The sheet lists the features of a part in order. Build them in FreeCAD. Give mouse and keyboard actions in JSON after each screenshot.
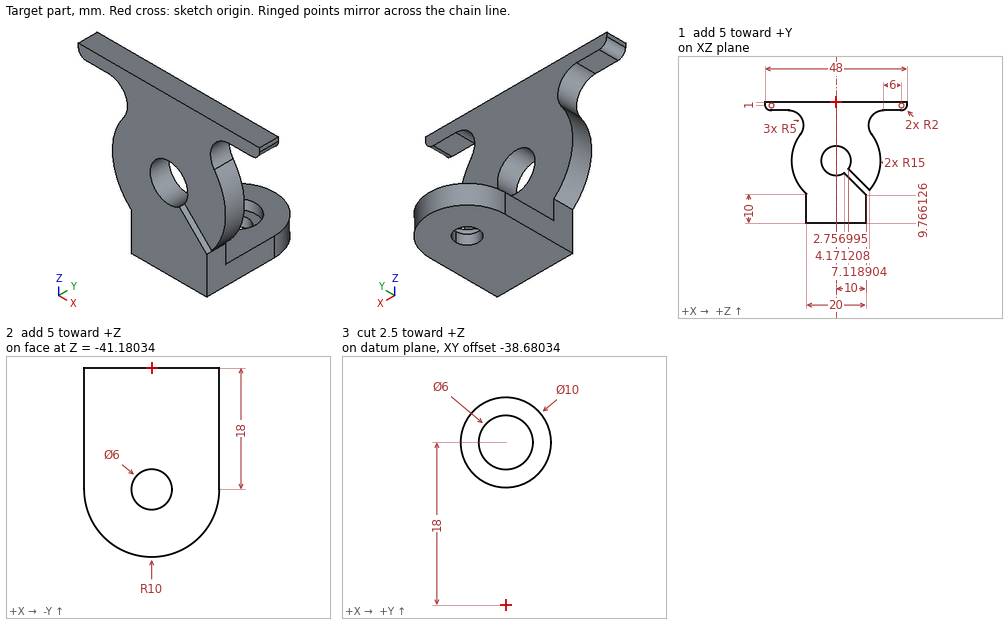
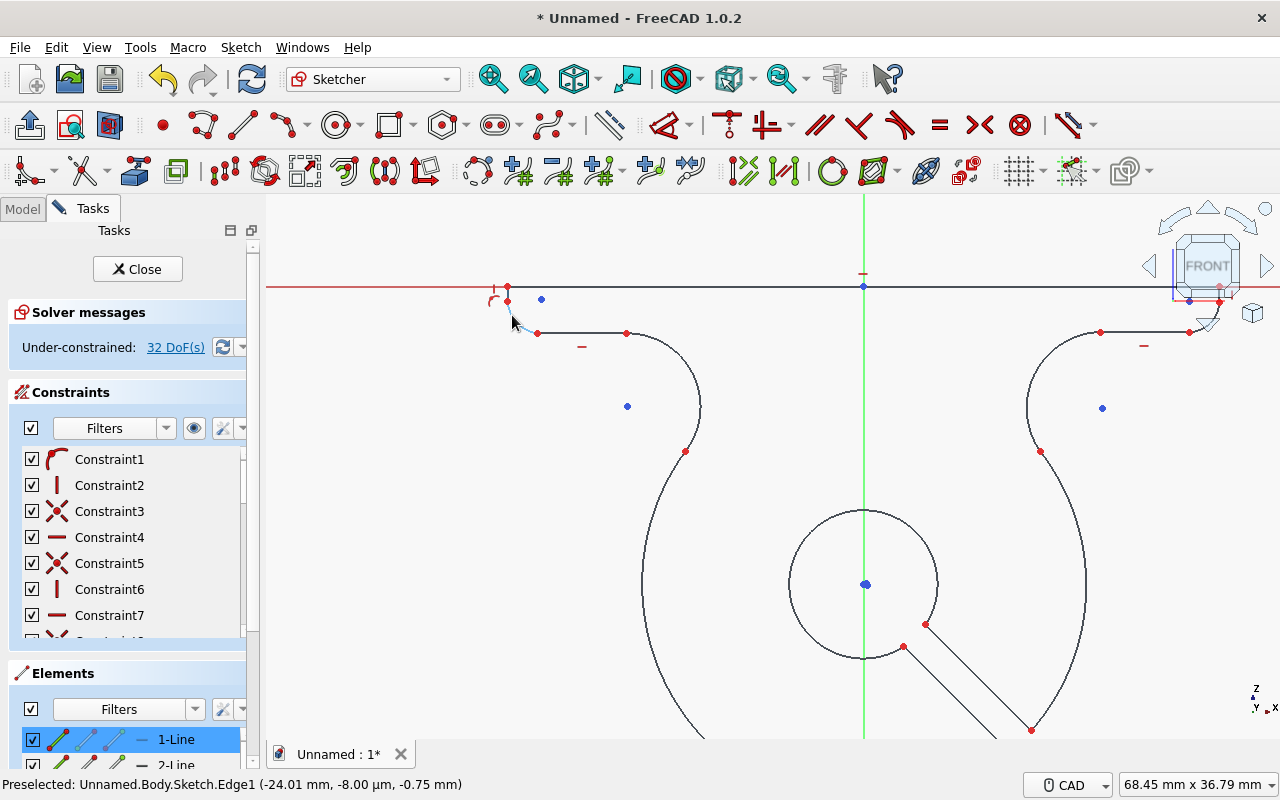
{"action": "left_click", "coordinate": [512, 315]}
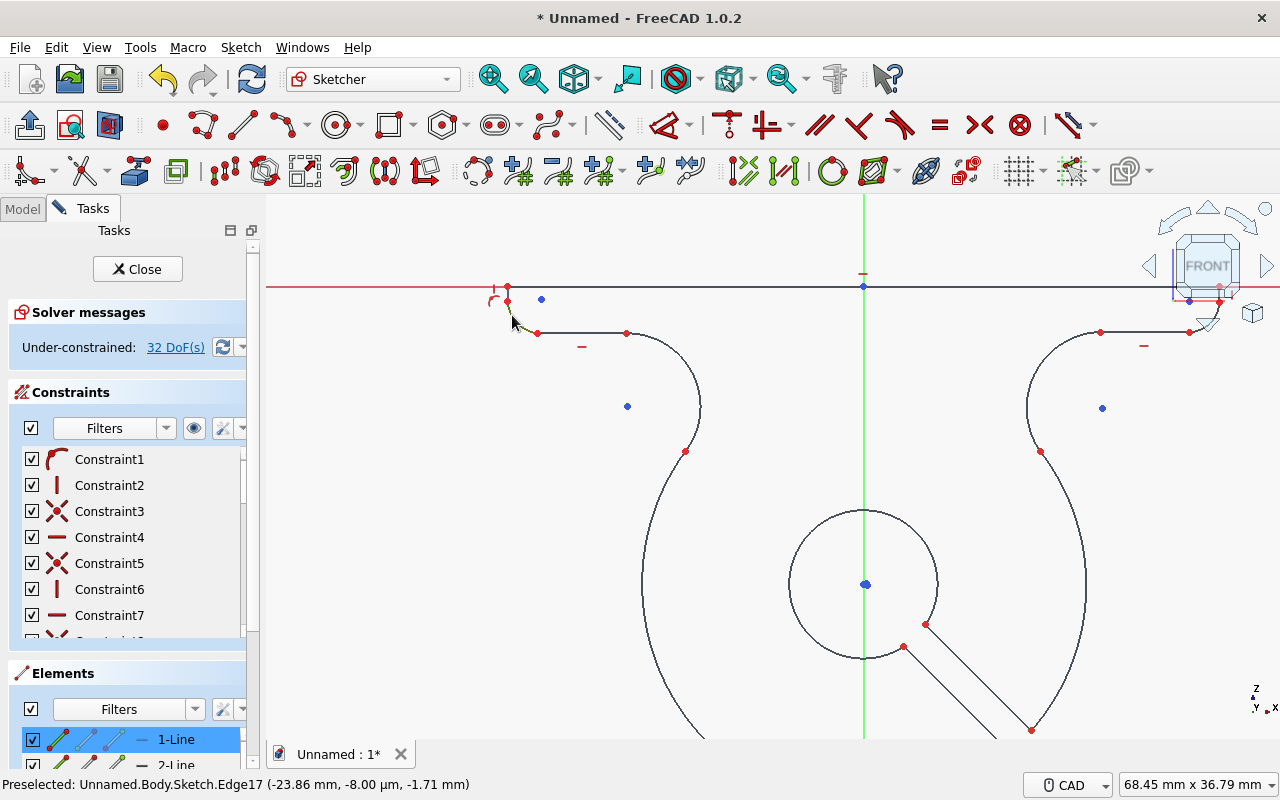
{"action": "key", "text": "t"}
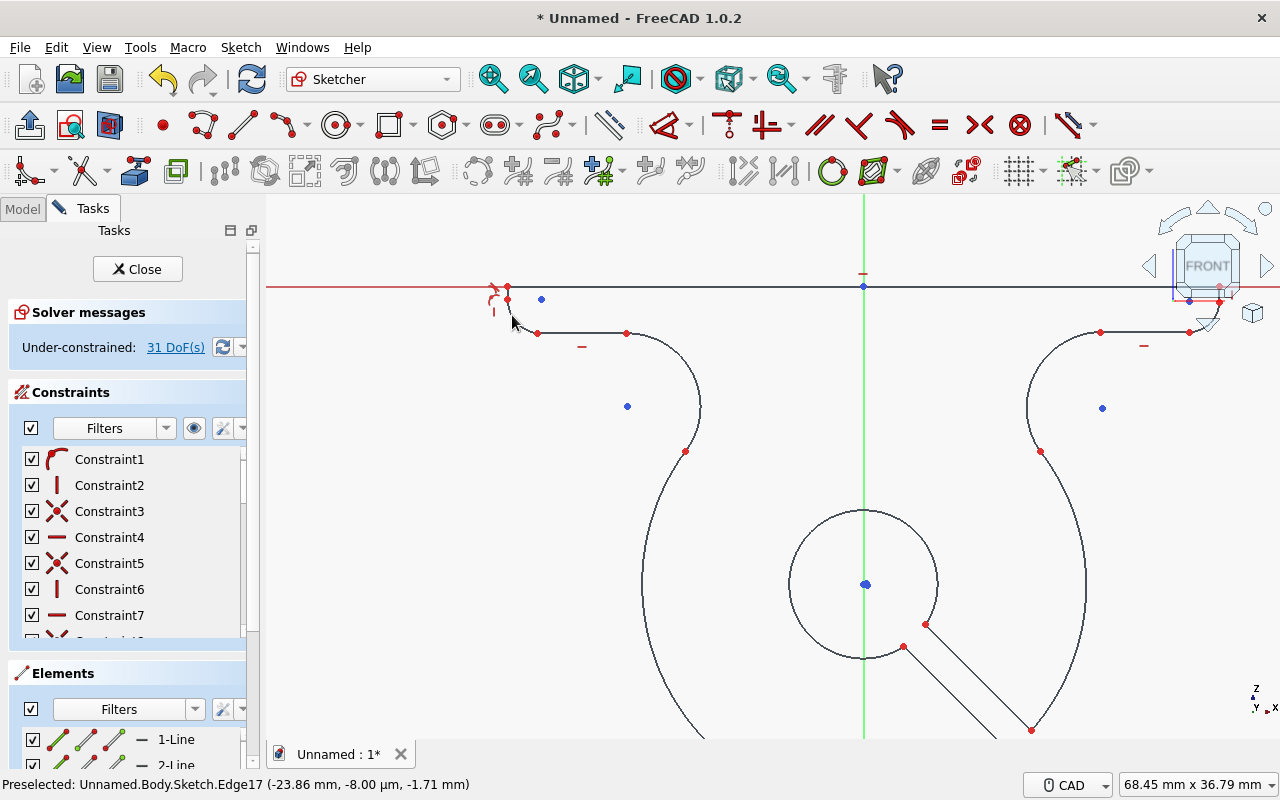
{"action": "scroll", "coordinate": [511, 314], "scroll_direction": "down", "scroll_amount": 3}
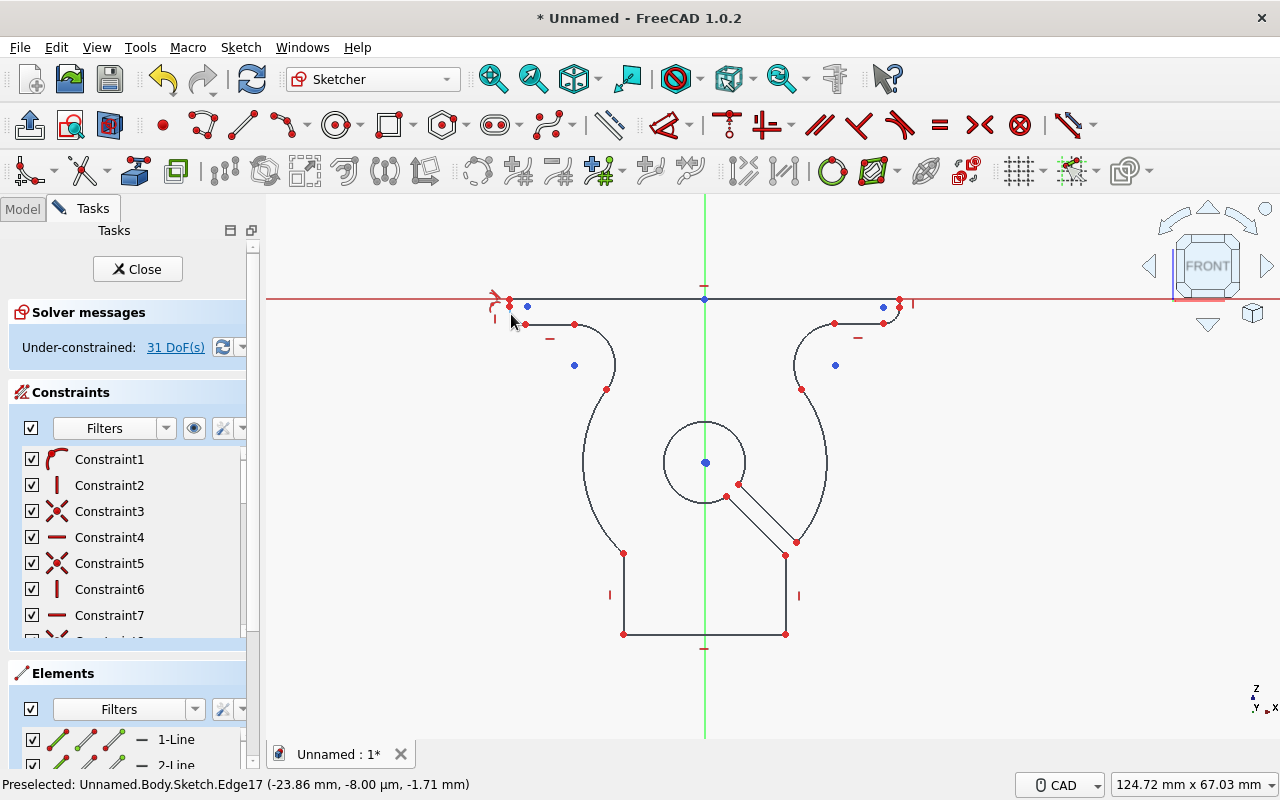
{"action": "scroll", "coordinate": [900, 303], "scroll_direction": "up", "scroll_amount": 6}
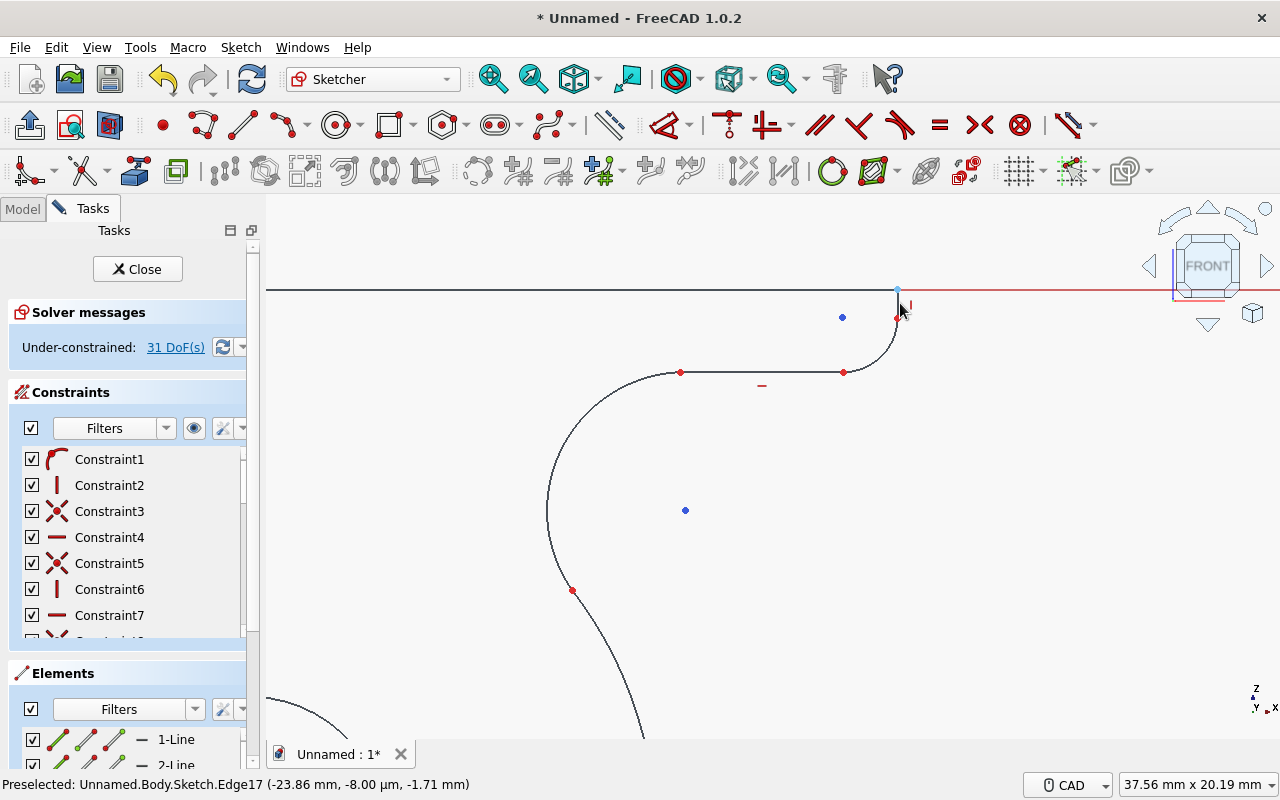
{"action": "left_click", "coordinate": [898, 304]}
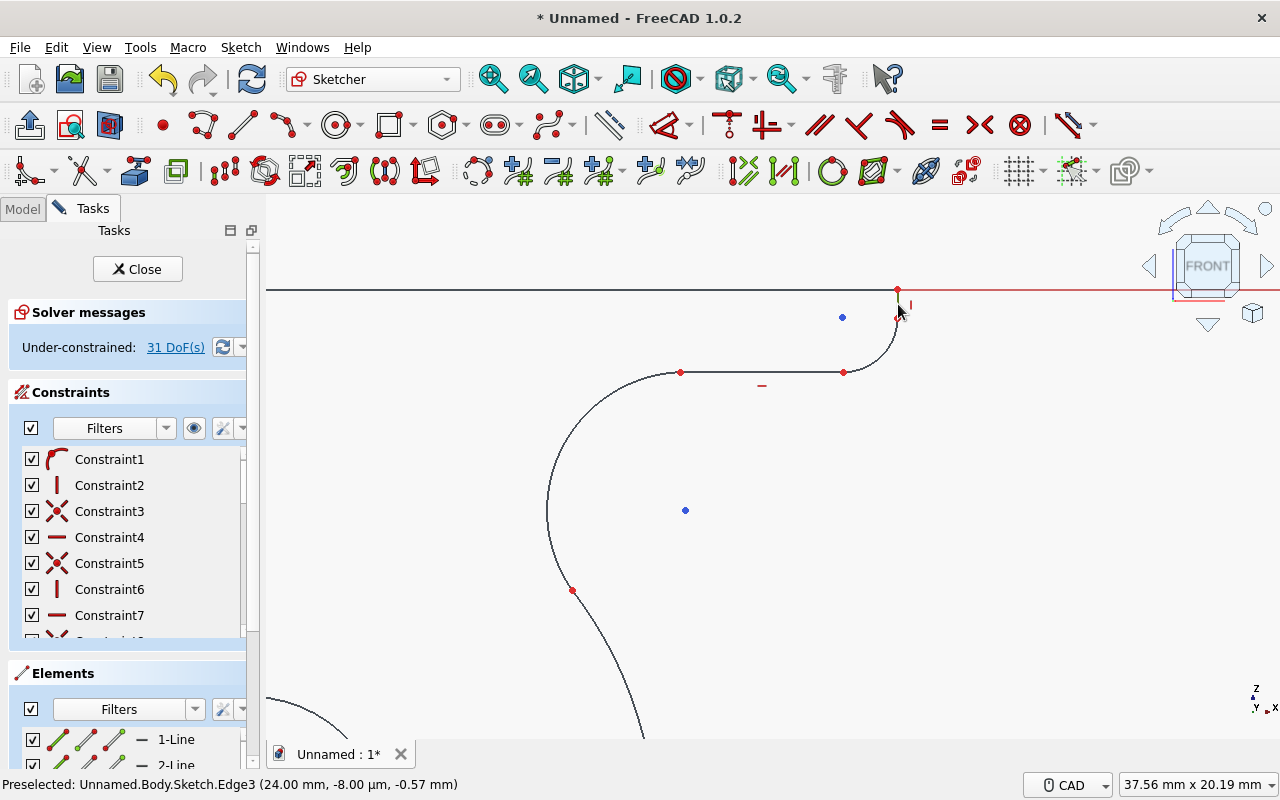
{"action": "left_click", "coordinate": [868, 366]}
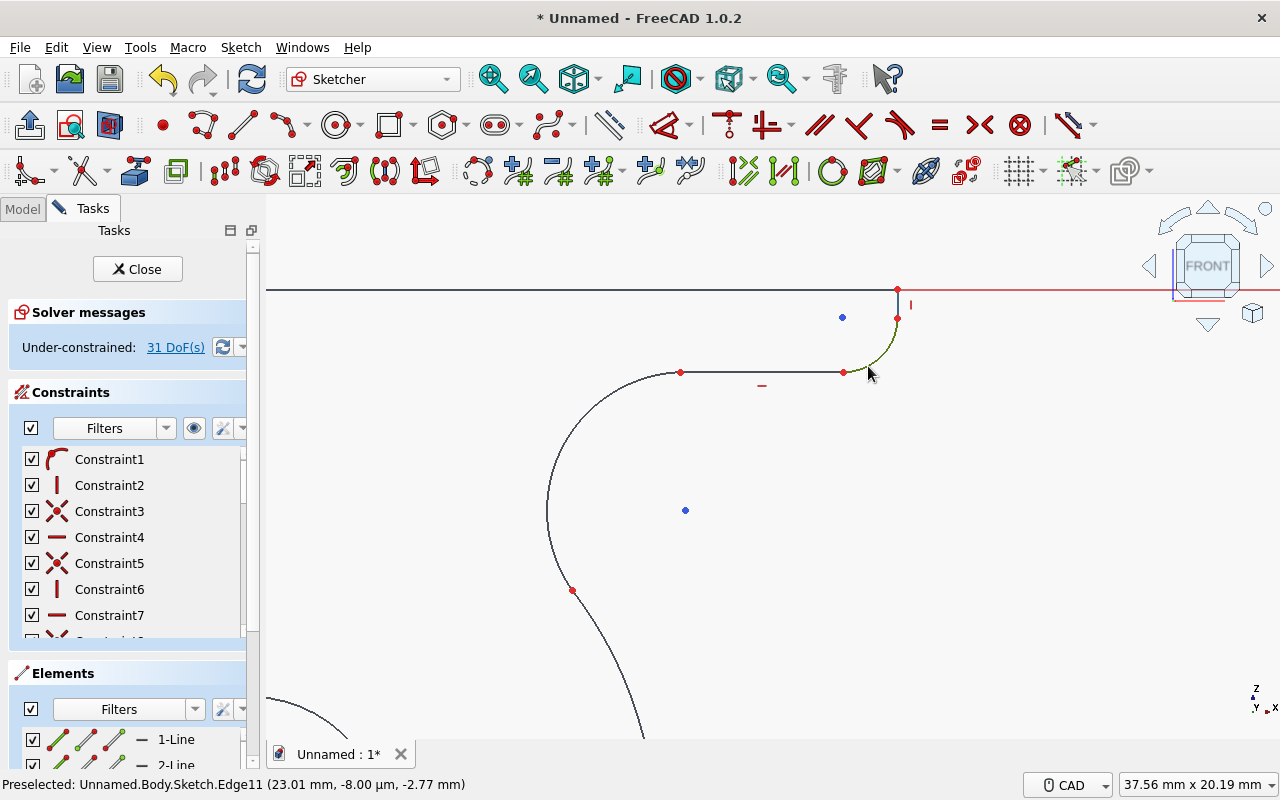
{"action": "key", "text": "t"}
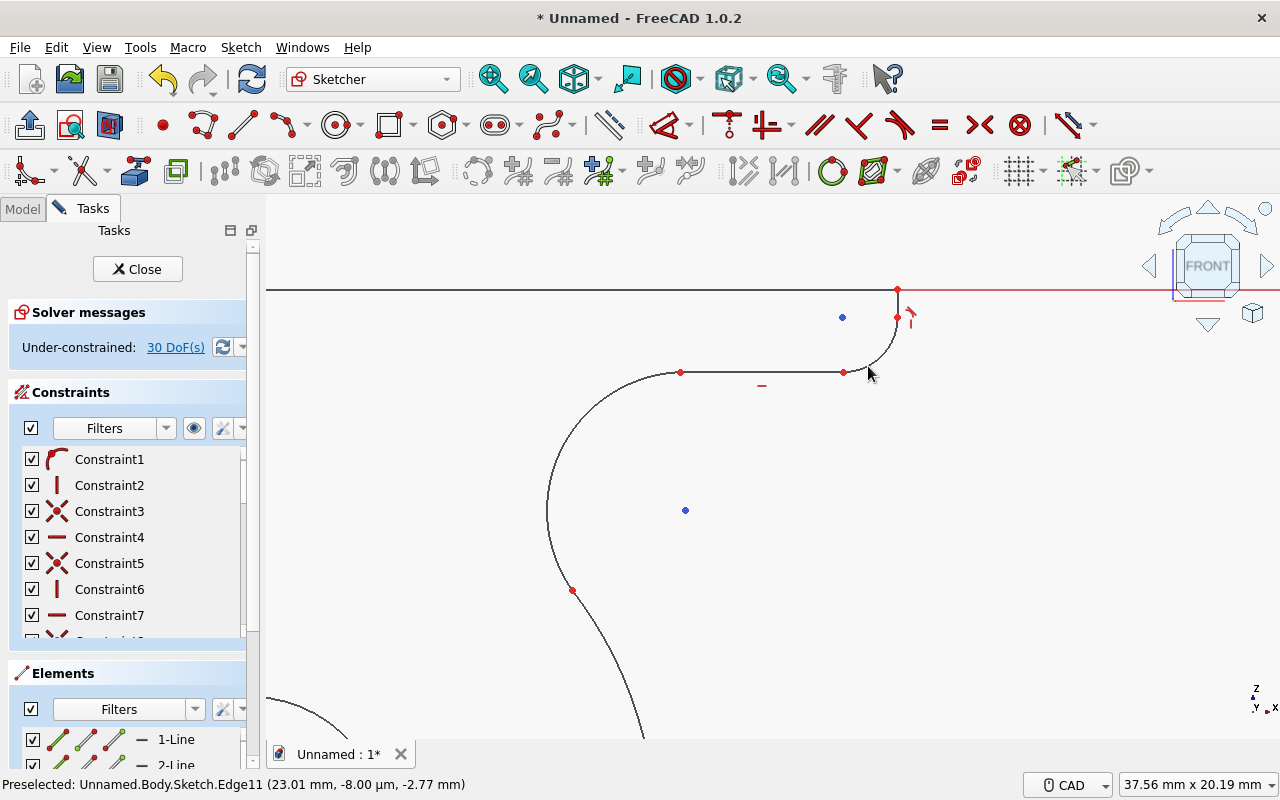
{"action": "left_click", "coordinate": [795, 372]}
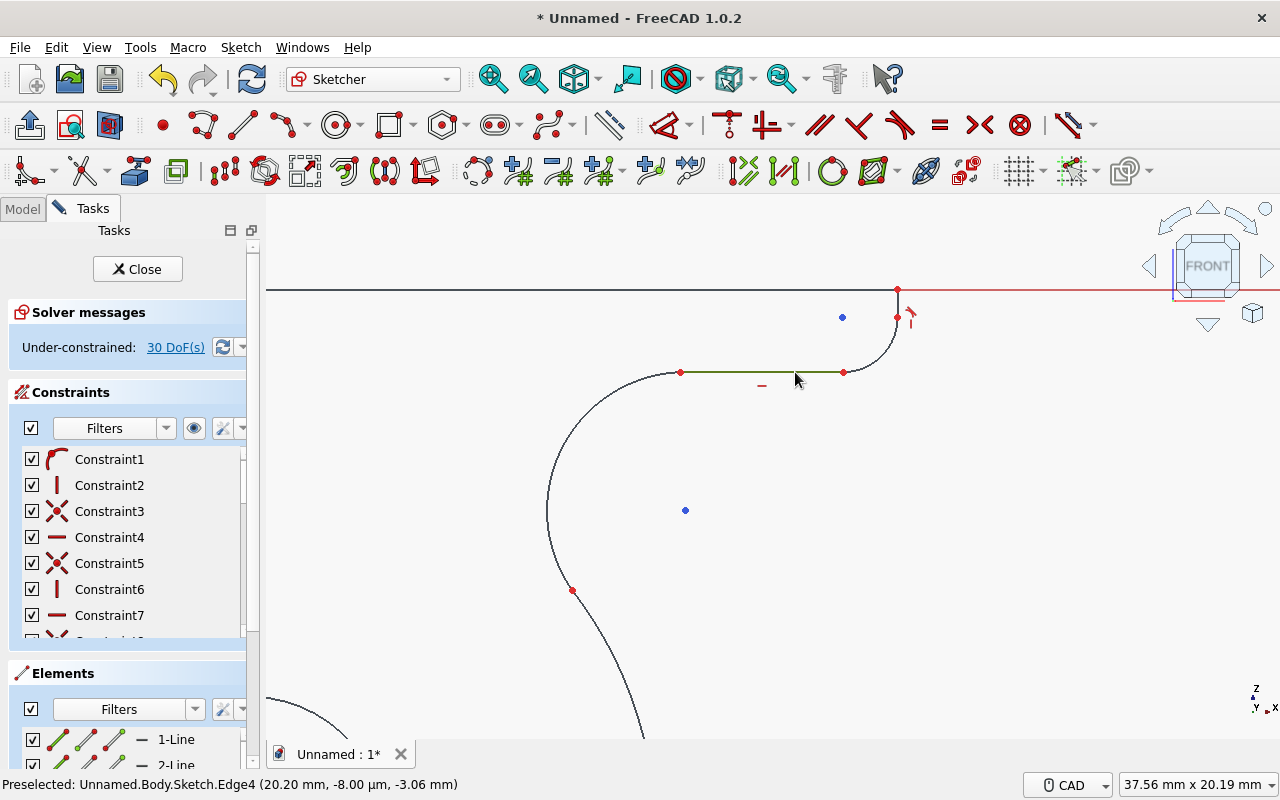
{"action": "left_click", "coordinate": [868, 366]}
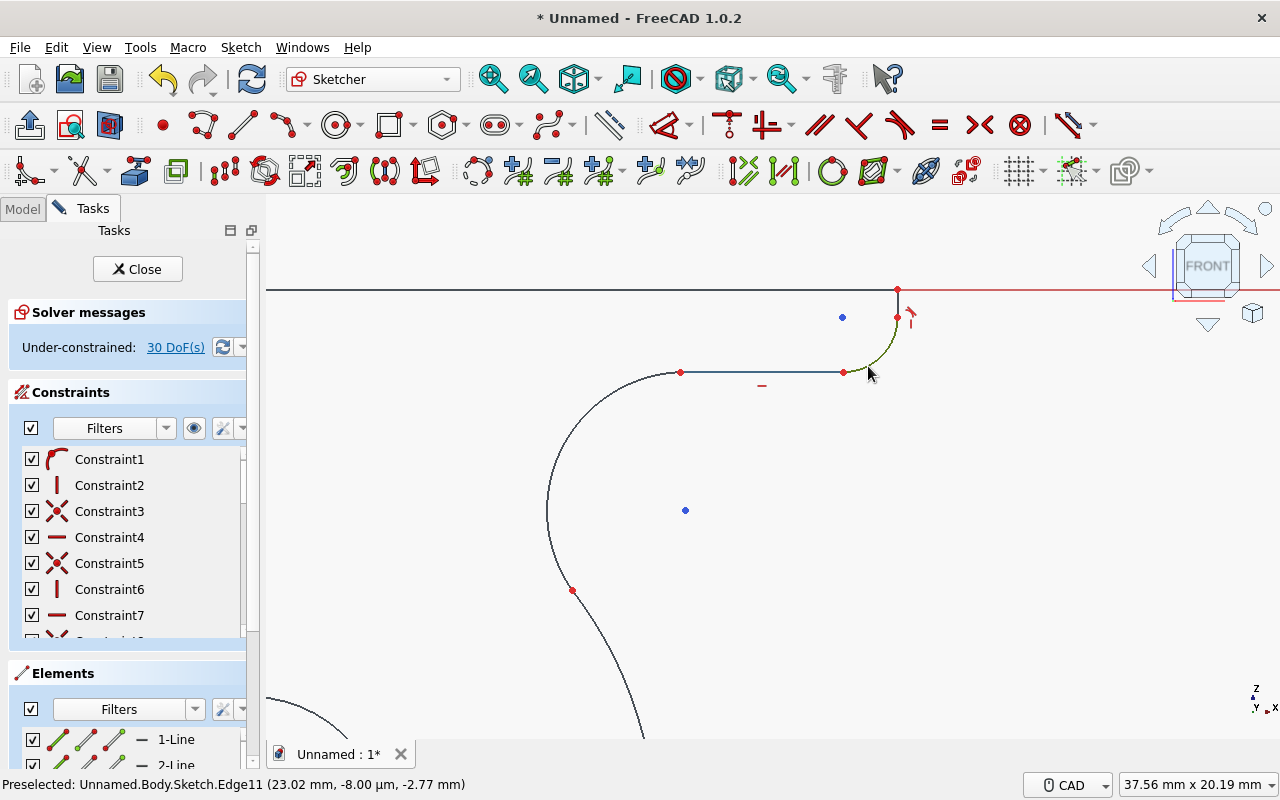
{"action": "key", "text": "t"}